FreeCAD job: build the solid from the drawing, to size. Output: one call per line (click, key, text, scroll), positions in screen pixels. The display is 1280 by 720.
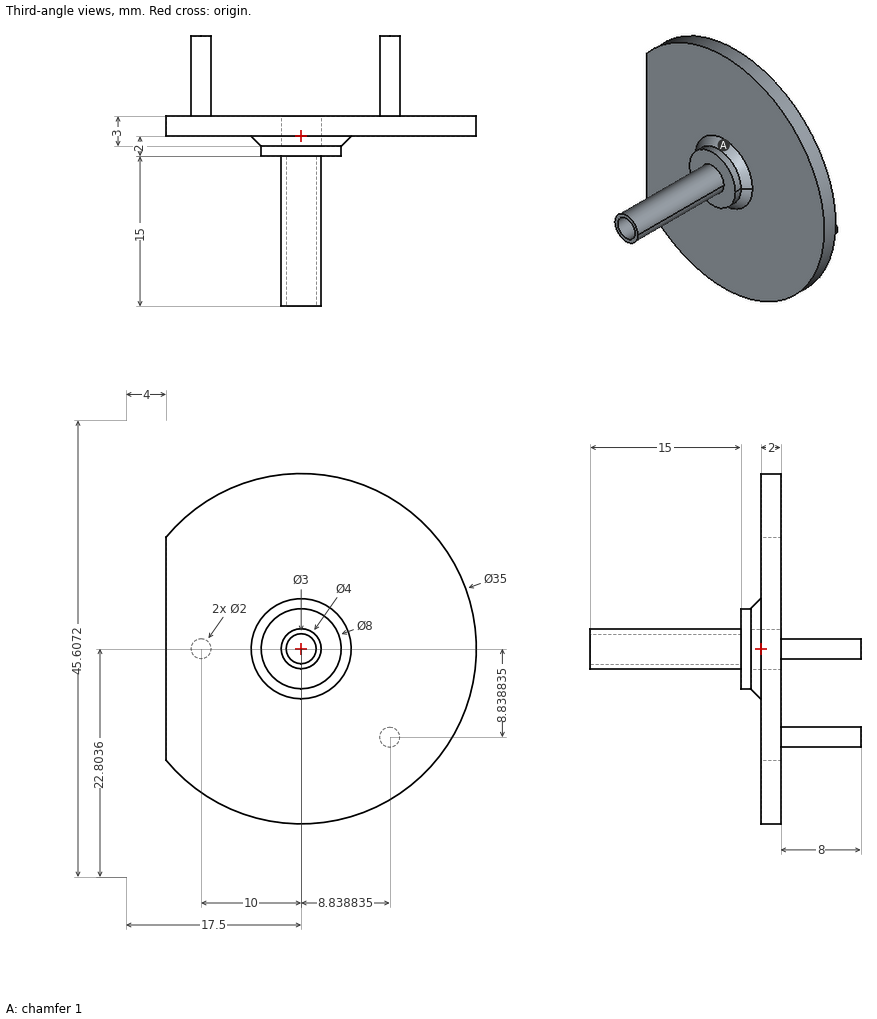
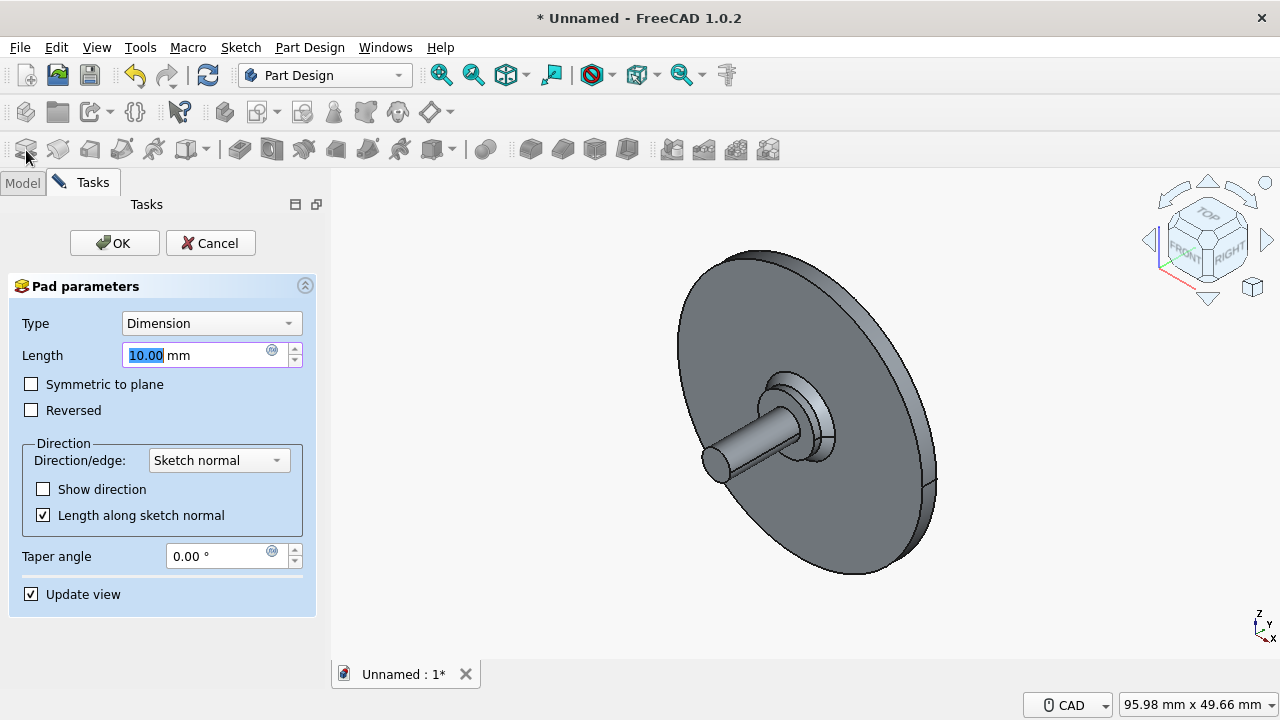
text(15)
key(Tab)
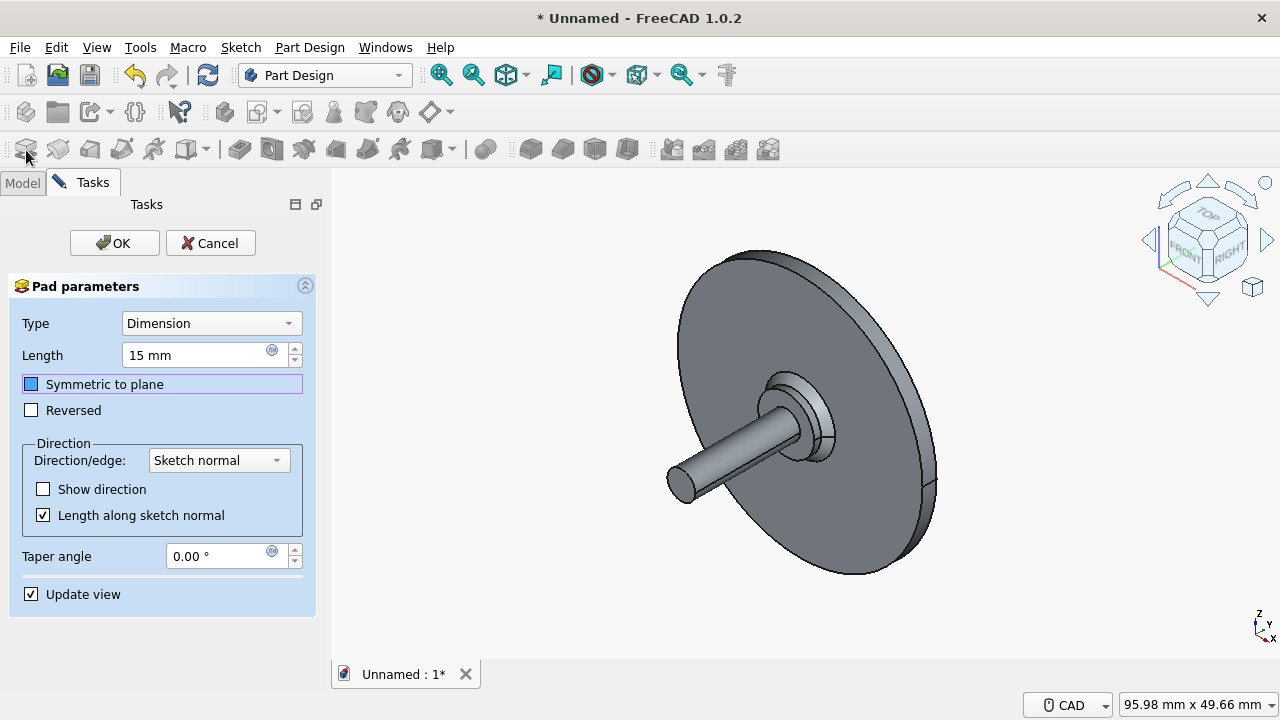
click(115, 243)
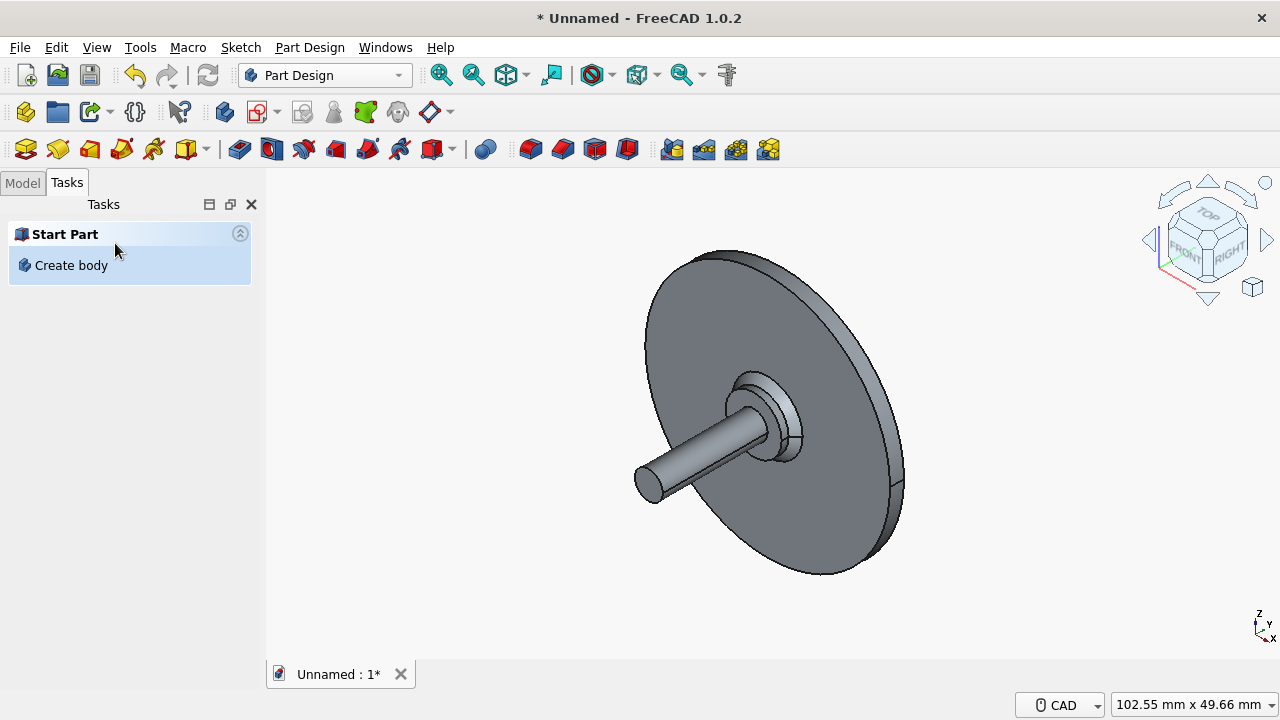
click(442, 76)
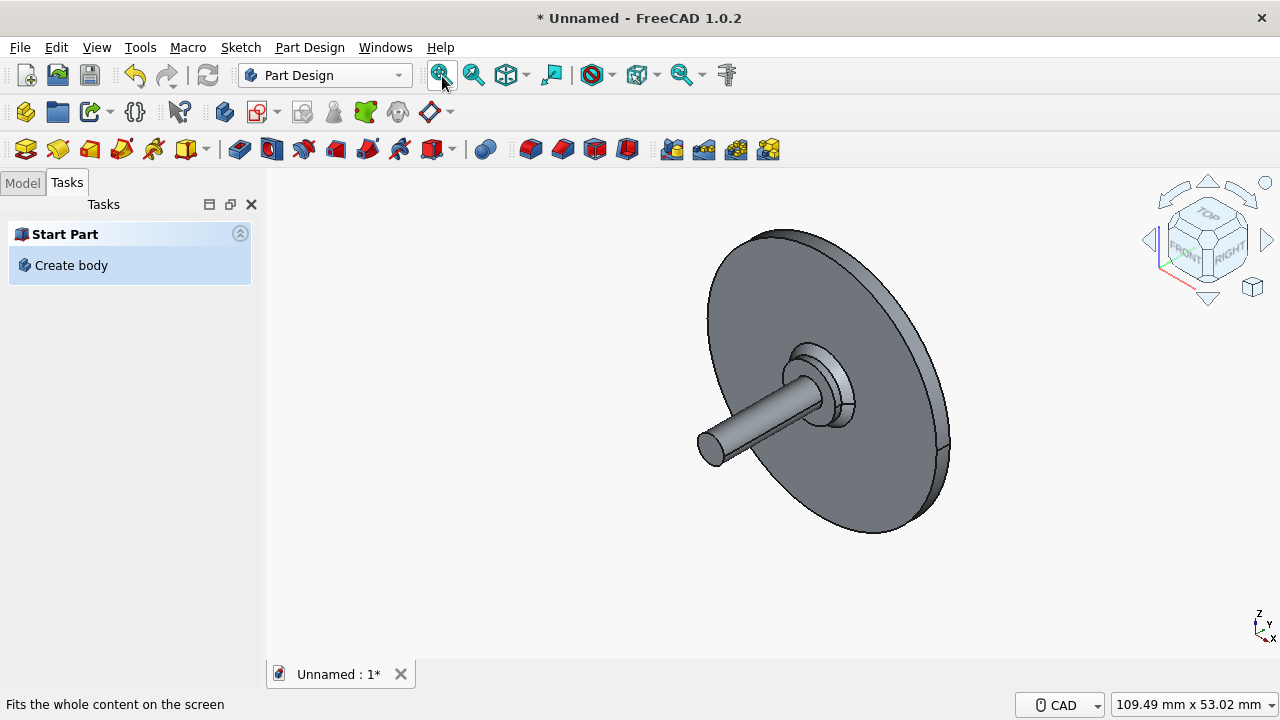
click(711, 448)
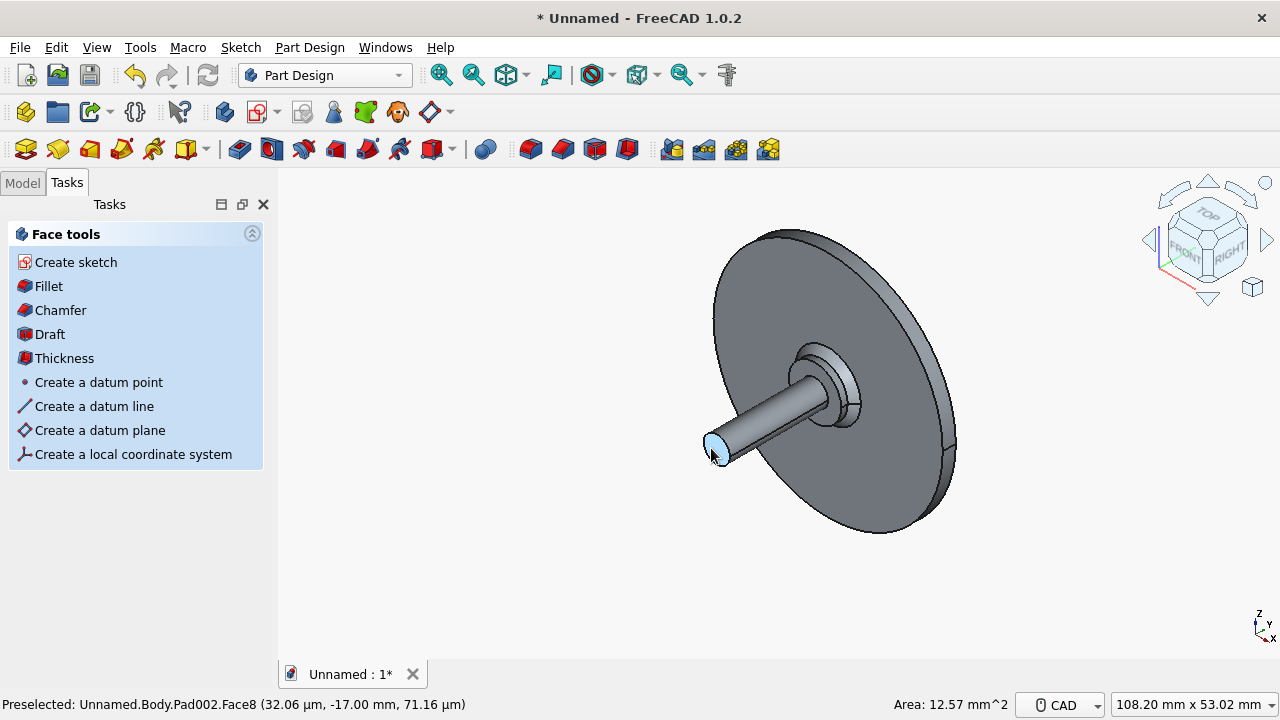
click(258, 112)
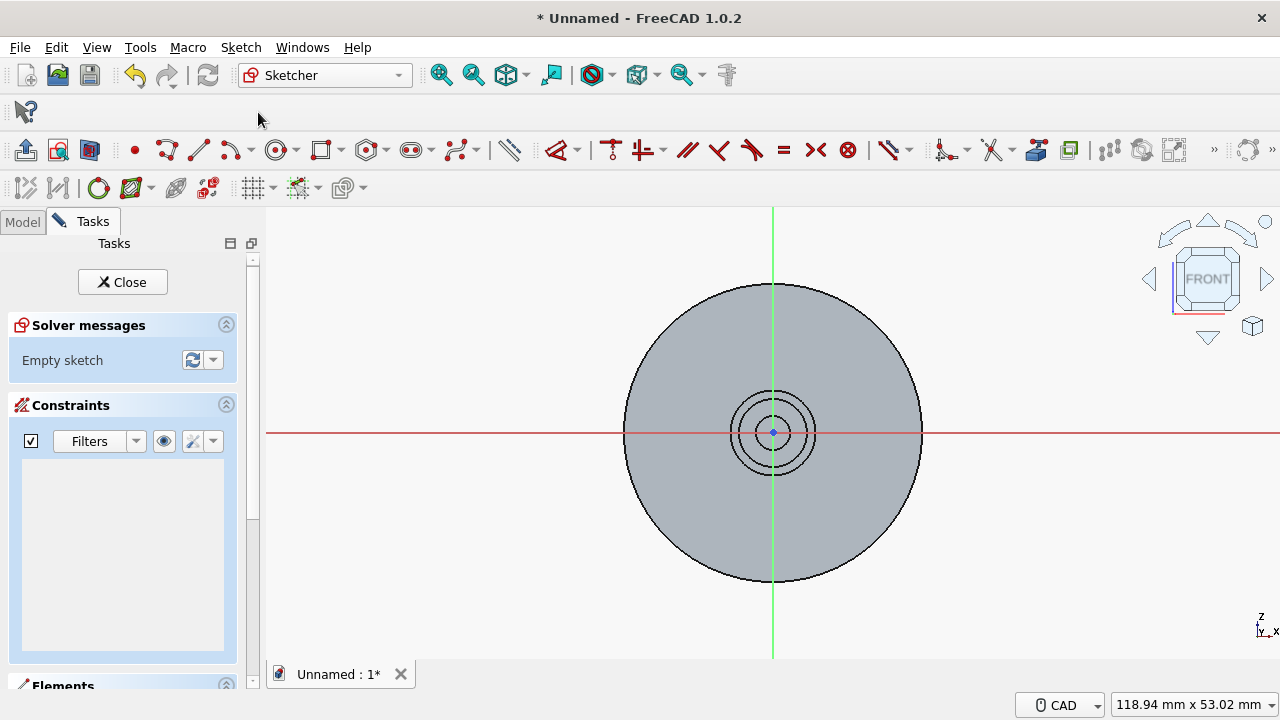
scroll(780, 433, up, 12)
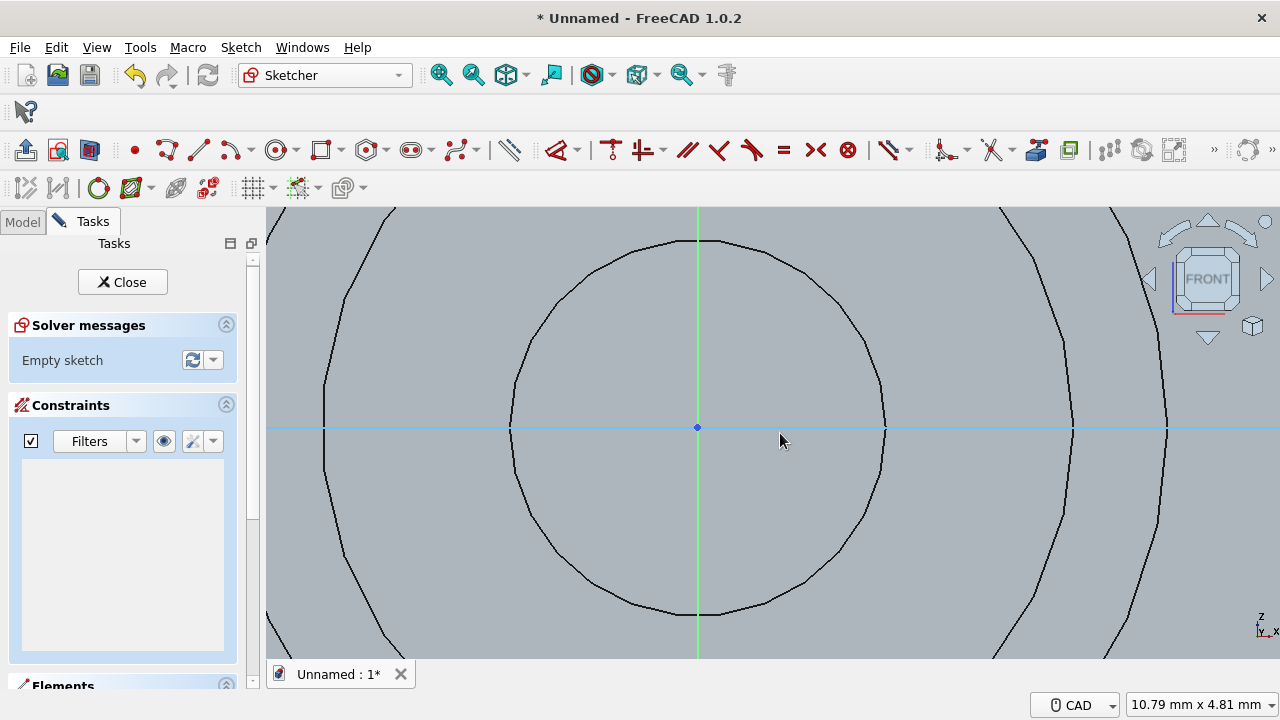
click(276, 150)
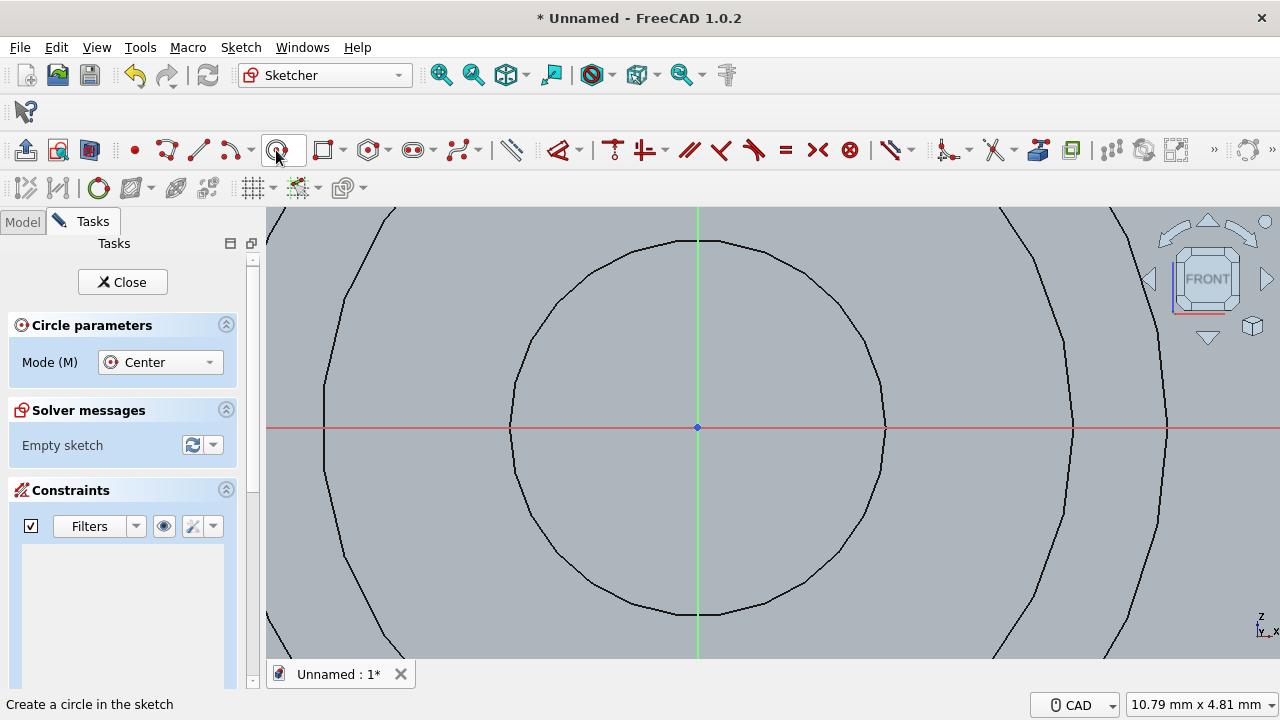
click(698, 428)
click(797, 328)
key(Escape)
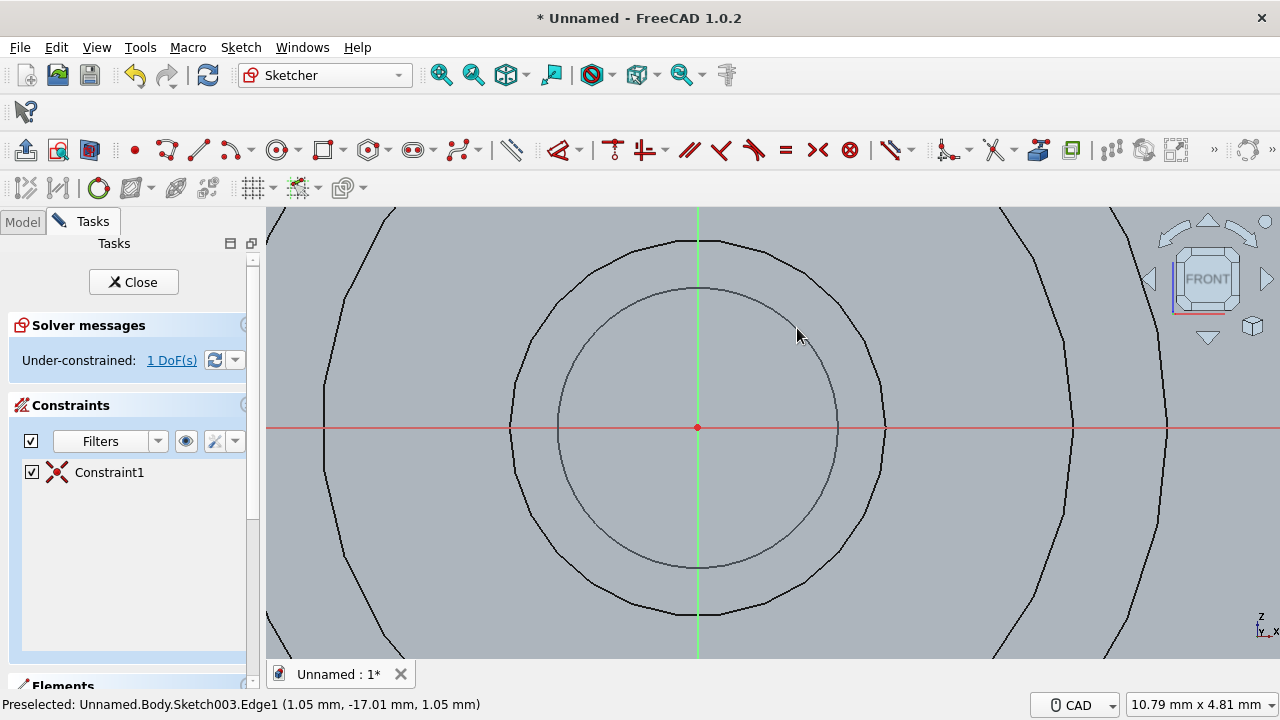
click(558, 150)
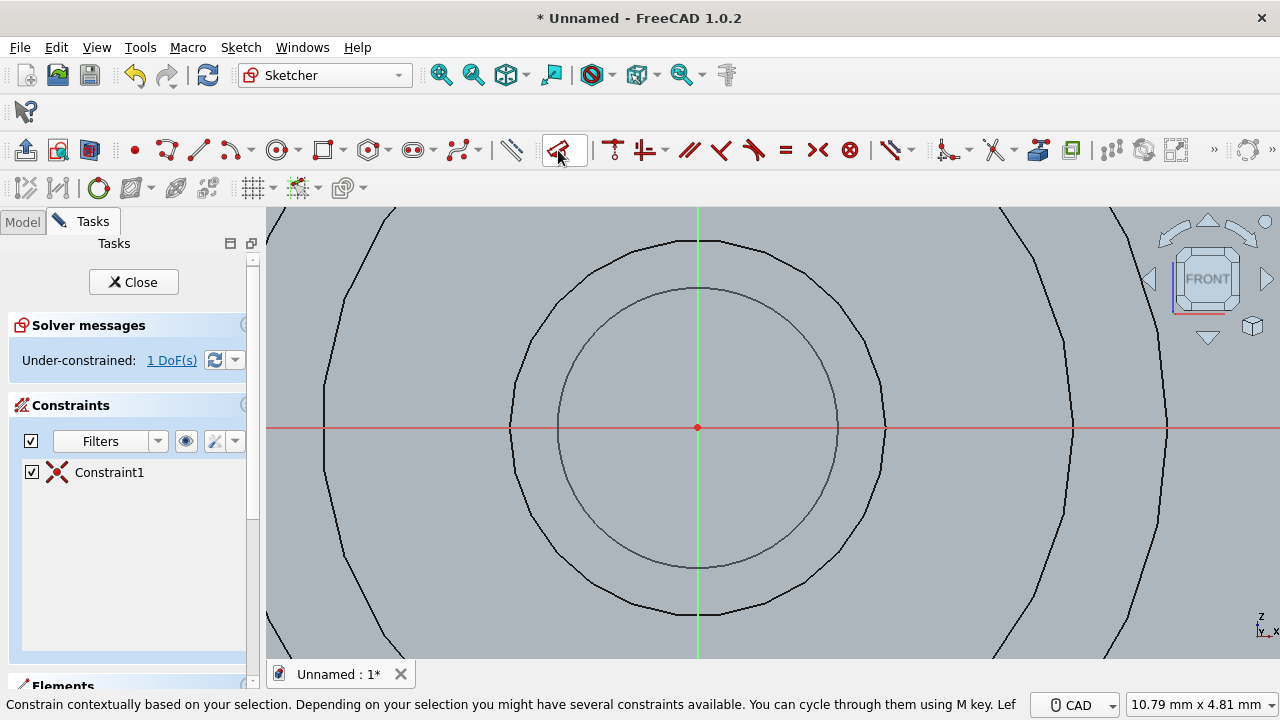
click(797, 329)
click(820, 306)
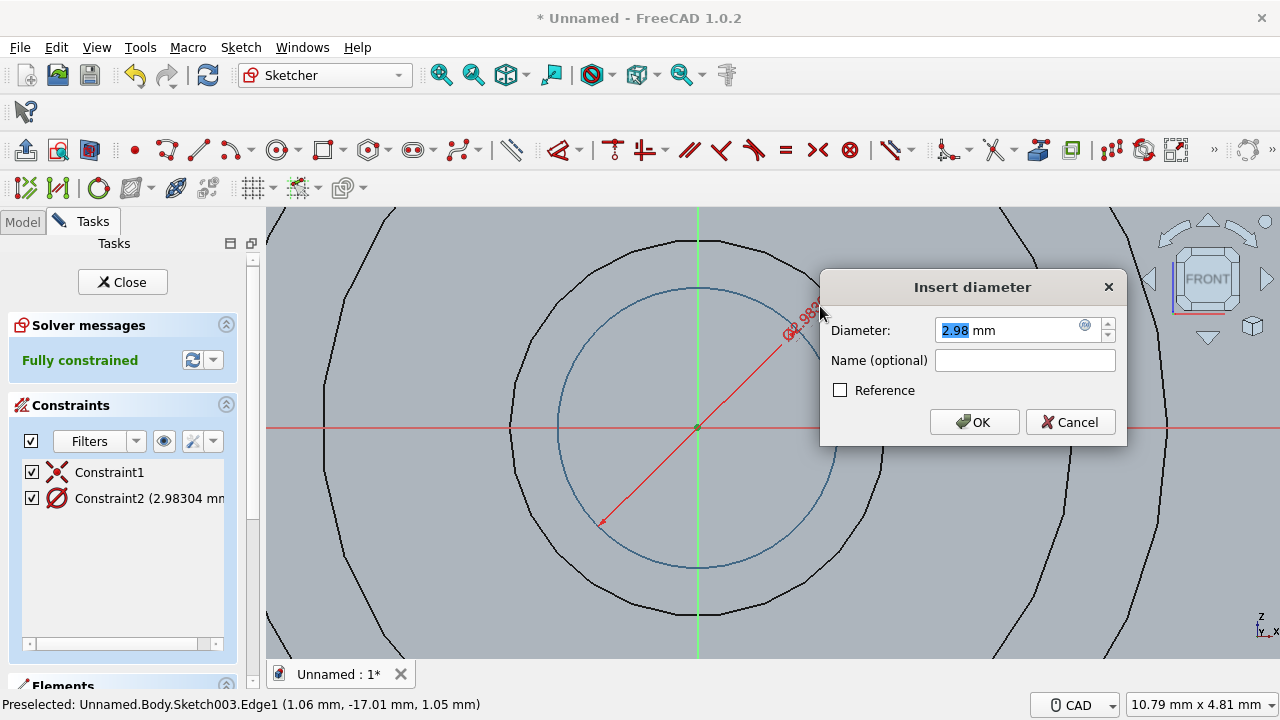
text(3)
key(Return)
key(Escape)